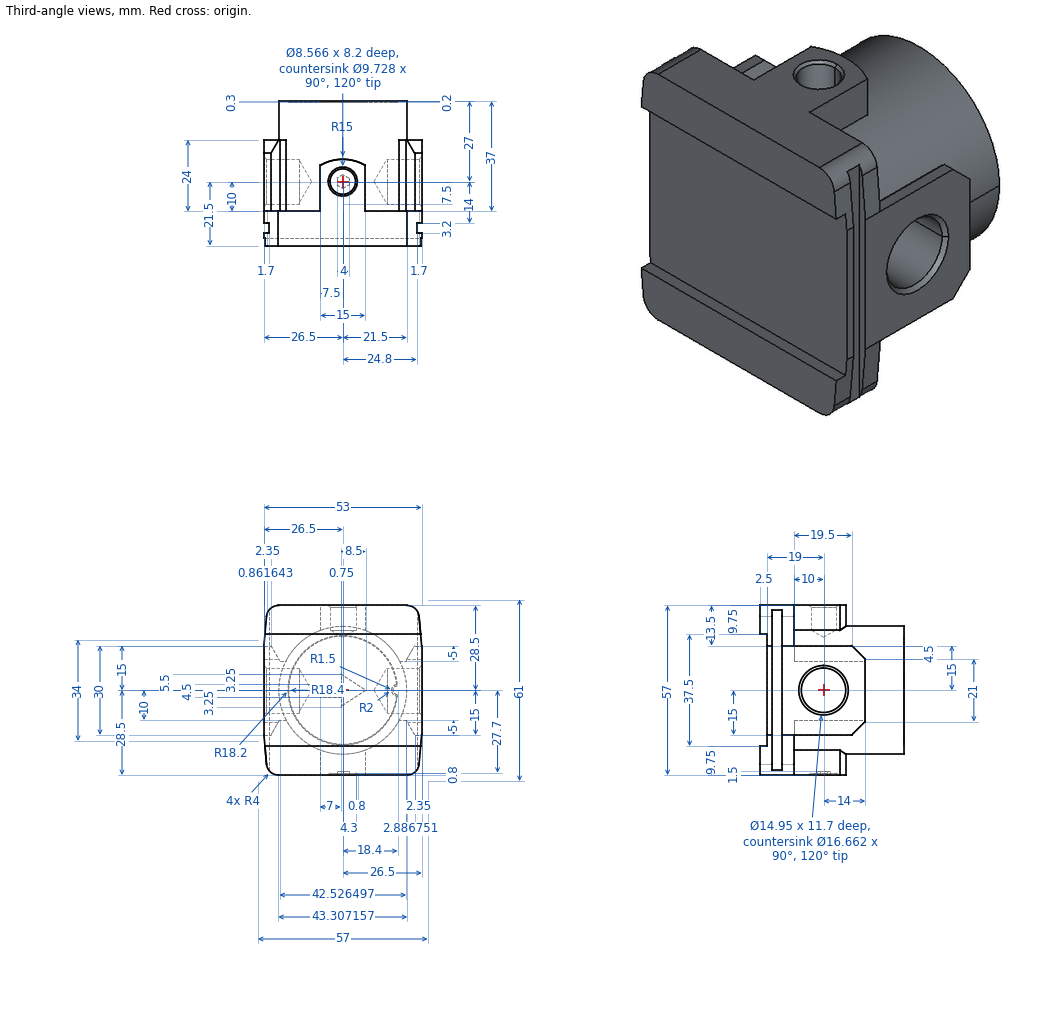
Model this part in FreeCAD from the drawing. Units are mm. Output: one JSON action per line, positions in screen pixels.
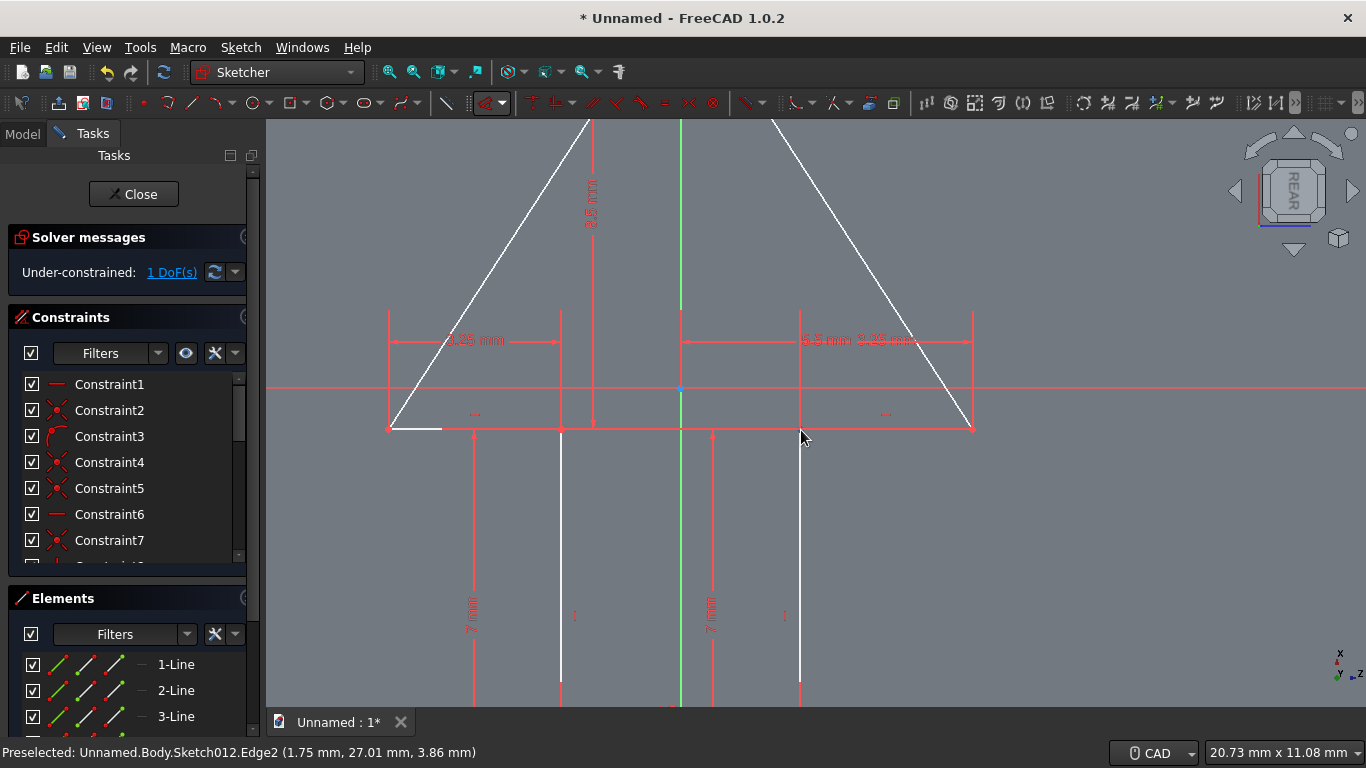
{"action": "left_click", "coordinate": [800, 429]}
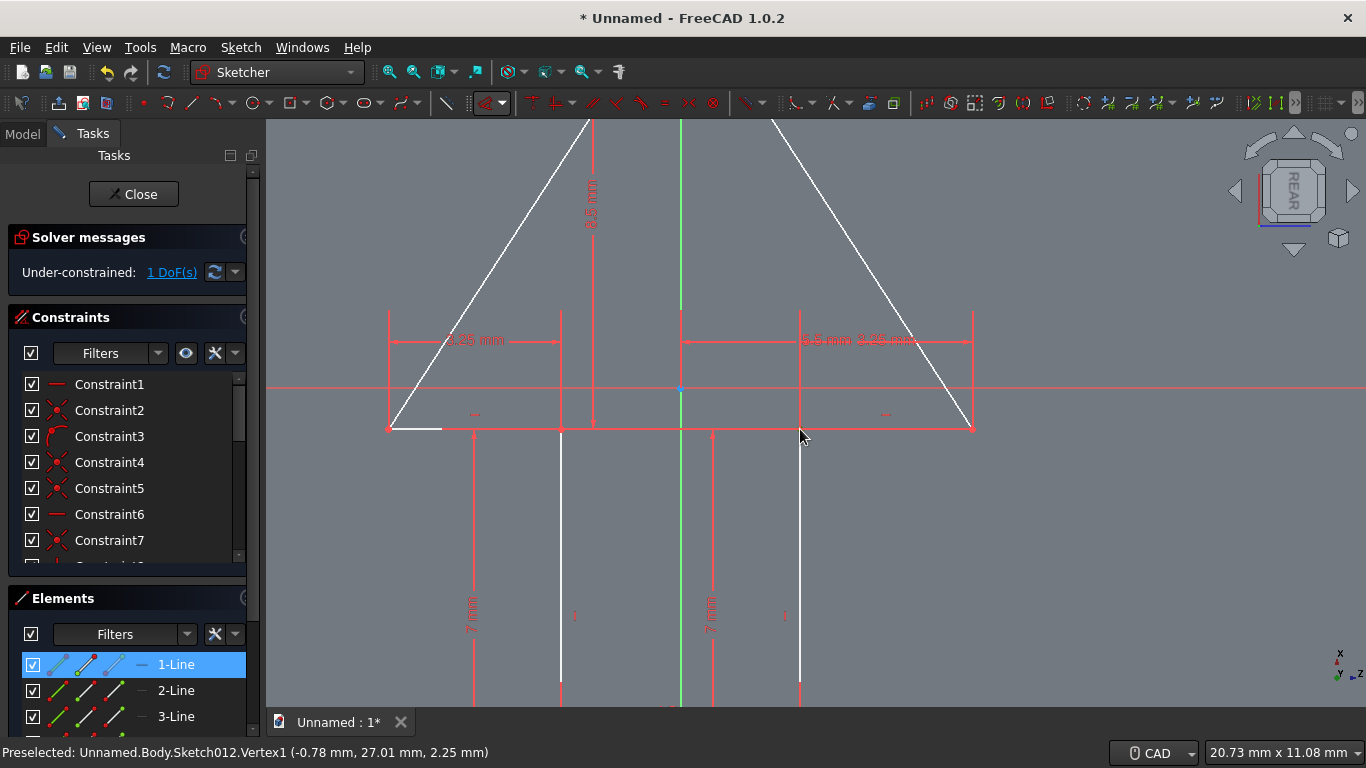
{"action": "left_click", "coordinate": [504, 104]}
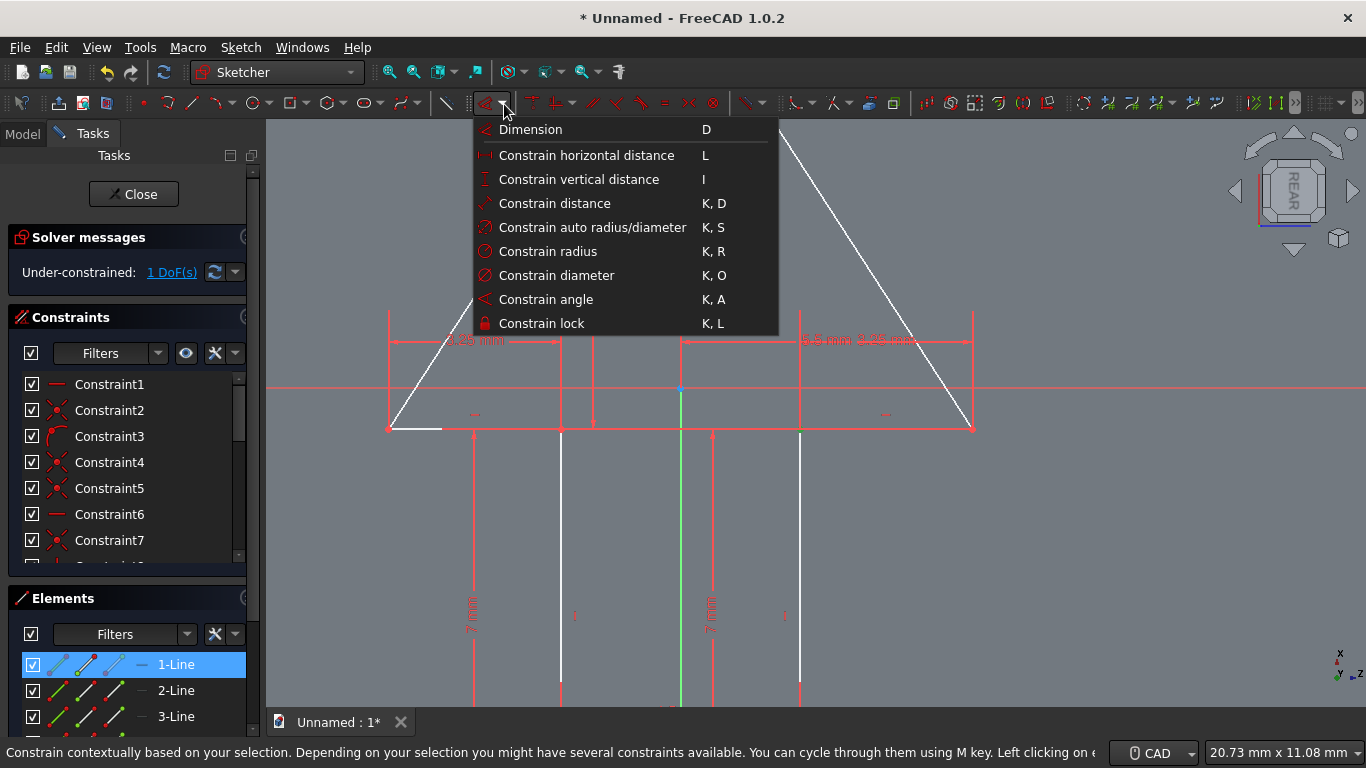
{"action": "left_click", "coordinate": [626, 179]}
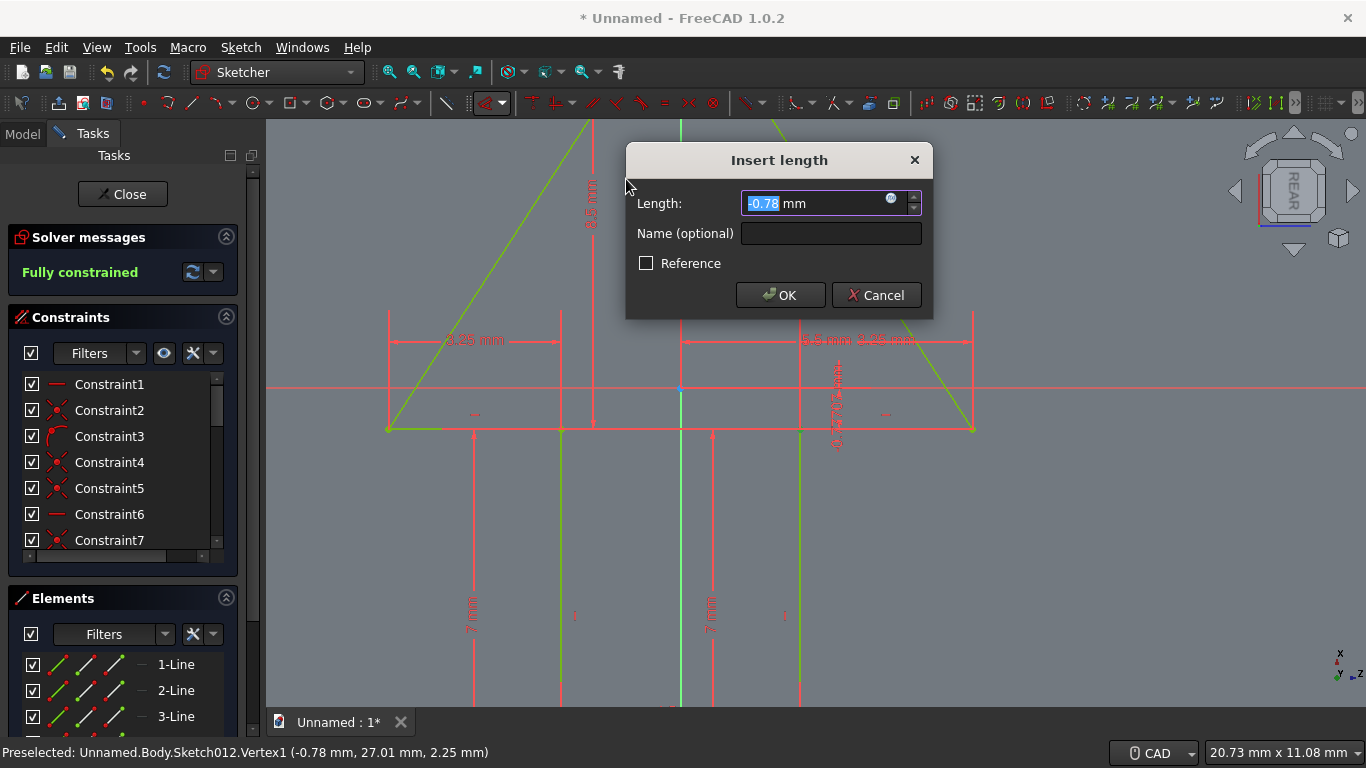
{"action": "type", "text": "-0.75"}
{"action": "key", "text": "Return"}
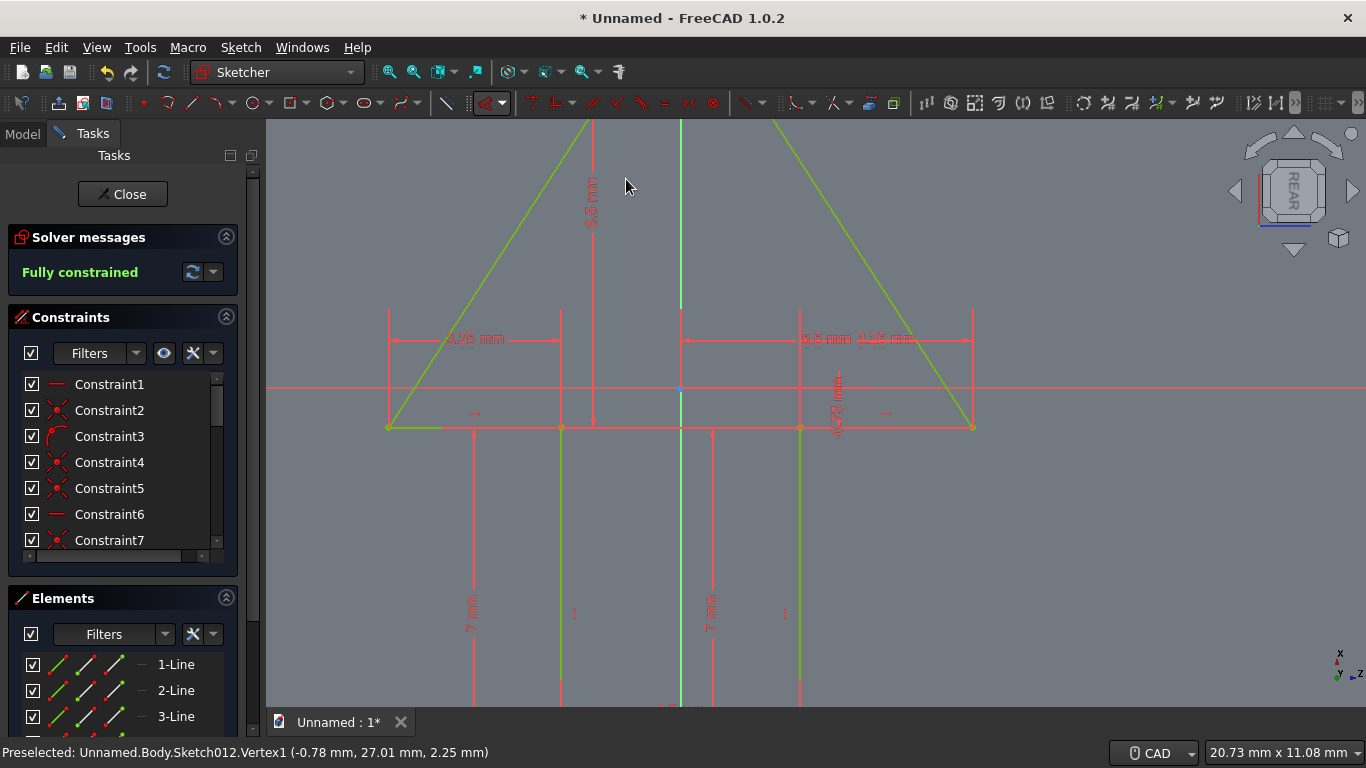
{"action": "left_click", "coordinate": [123, 194]}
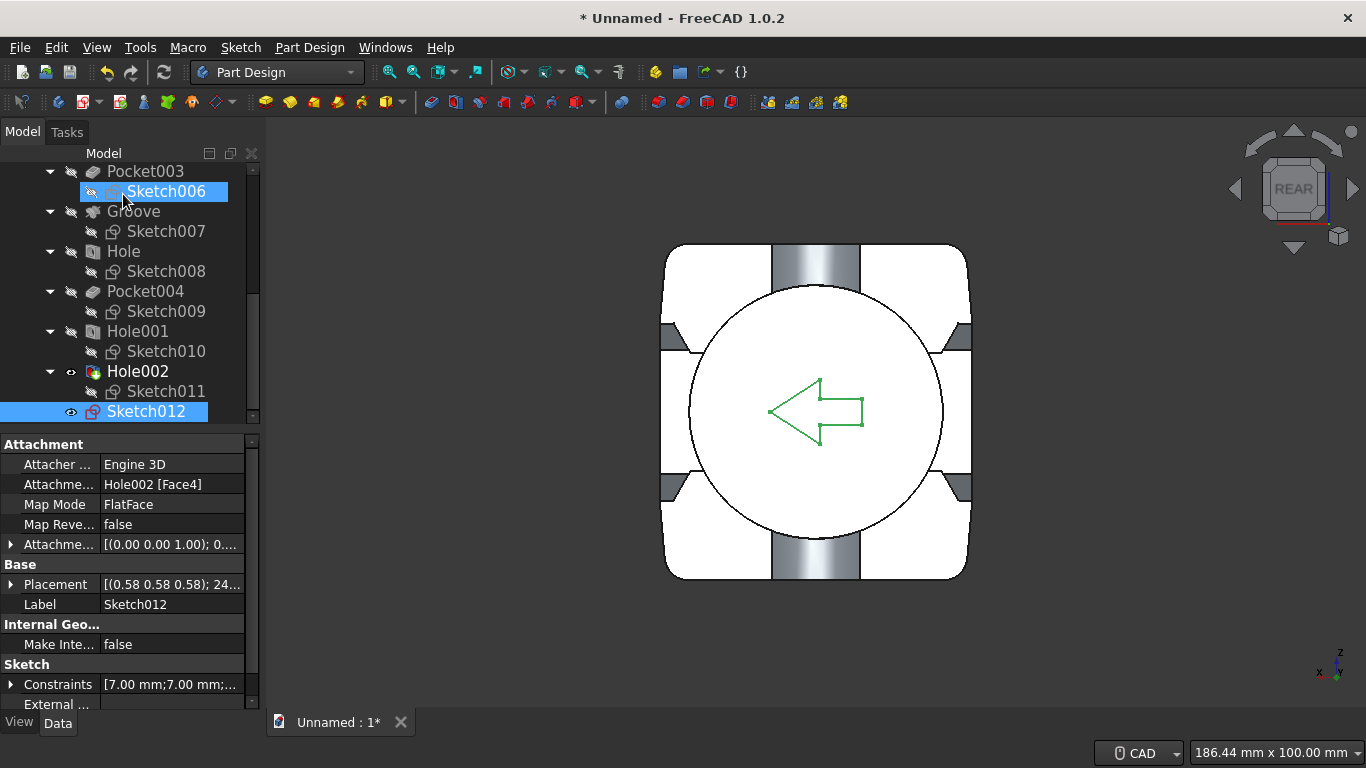
{"action": "left_click", "coordinate": [432, 102]}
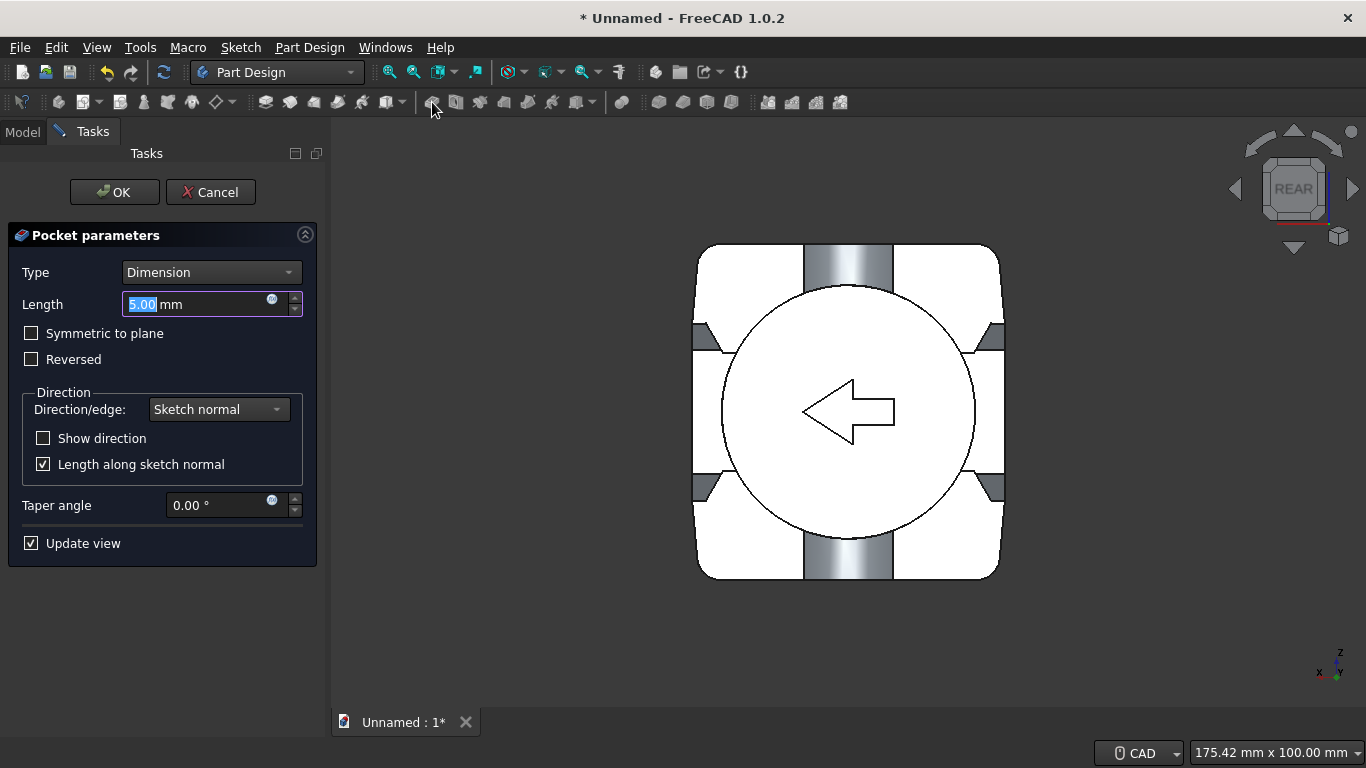
{"action": "type", "text": "0.3"}
{"action": "key", "text": "Tab"}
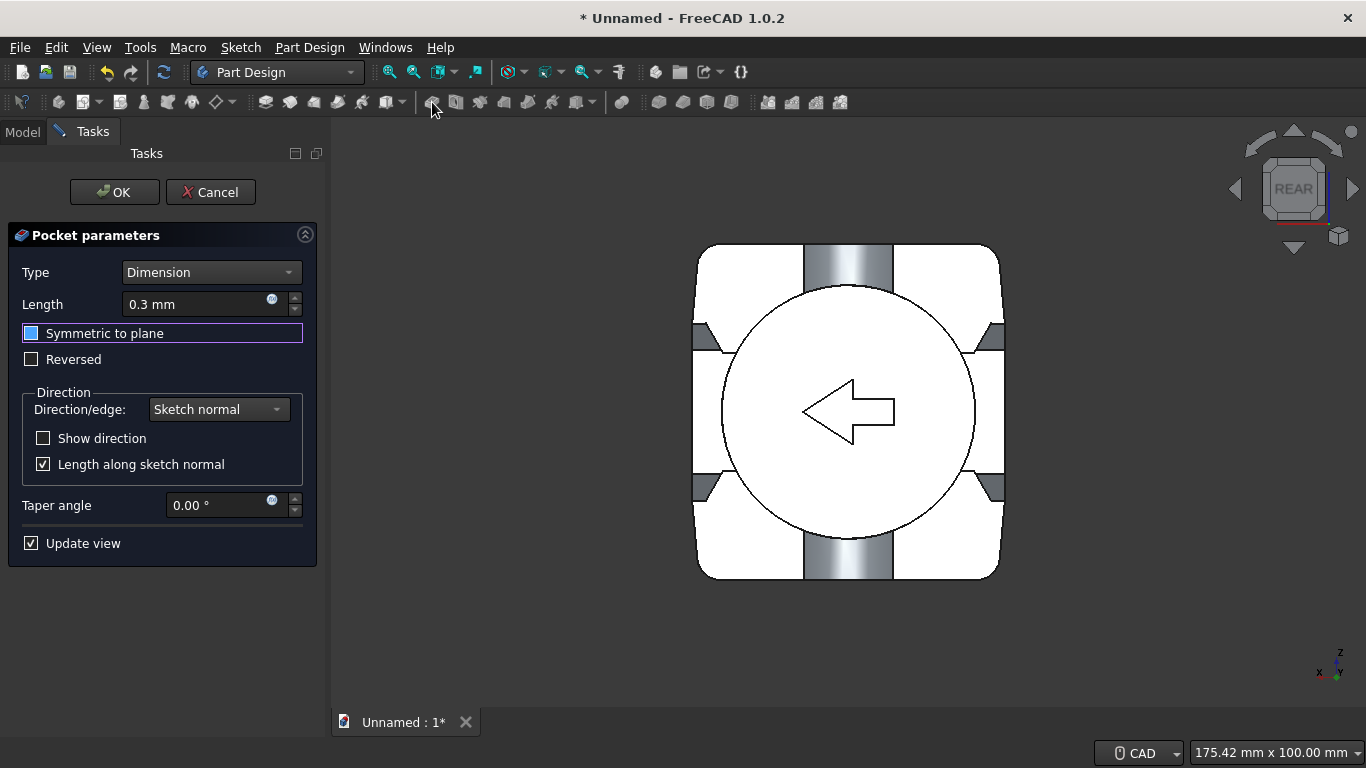
{"action": "left_click", "coordinate": [115, 192]}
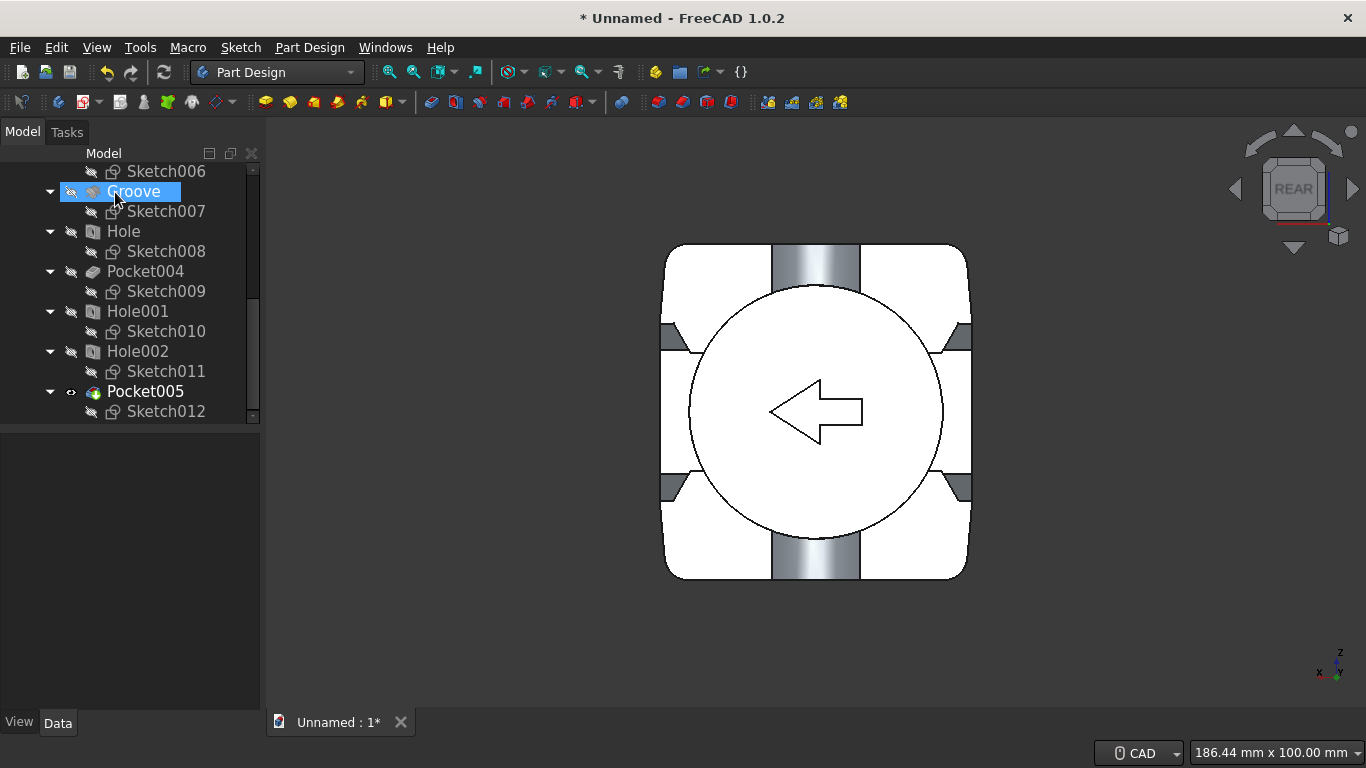
{"action": "left_click", "coordinate": [780, 483]}